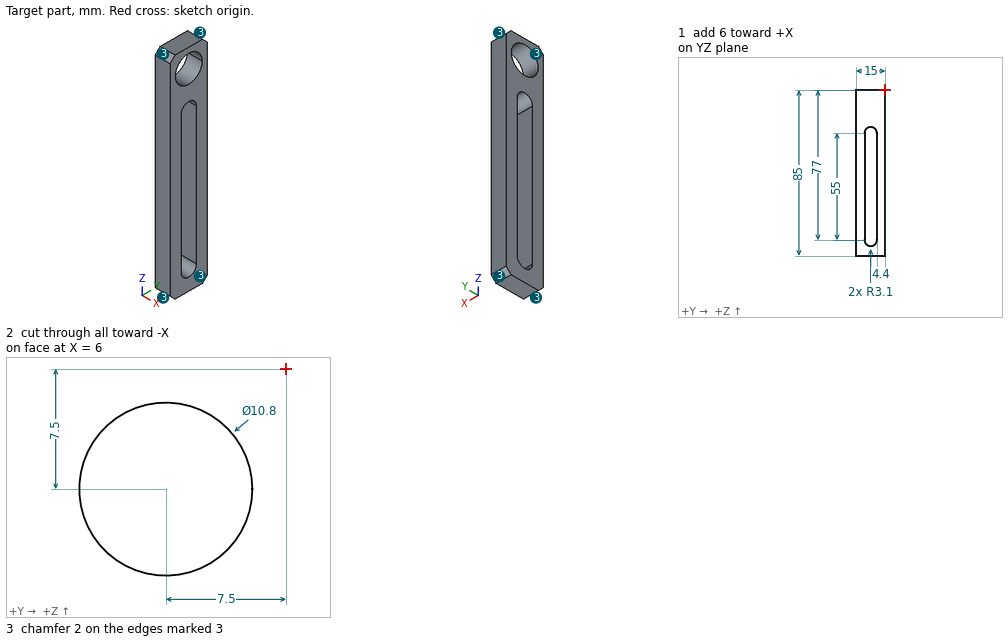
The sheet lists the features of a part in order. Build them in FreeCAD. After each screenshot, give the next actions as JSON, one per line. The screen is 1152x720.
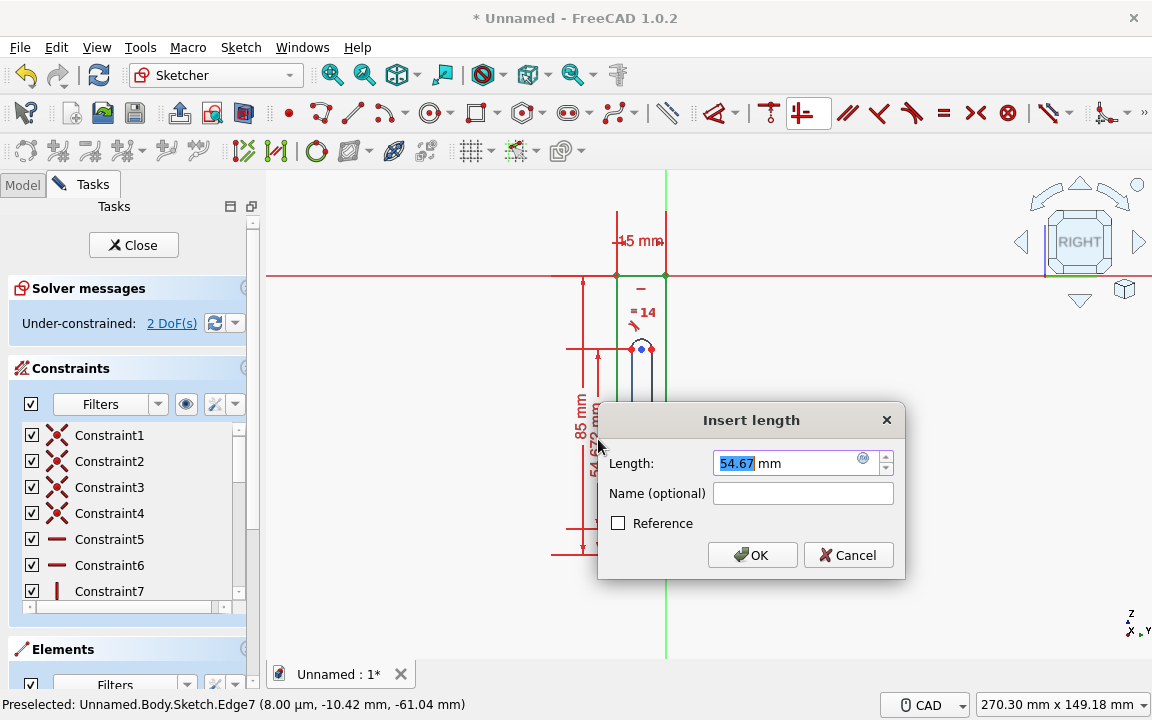
{"action": "type", "text": "55"}
{"action": "key", "text": "Return"}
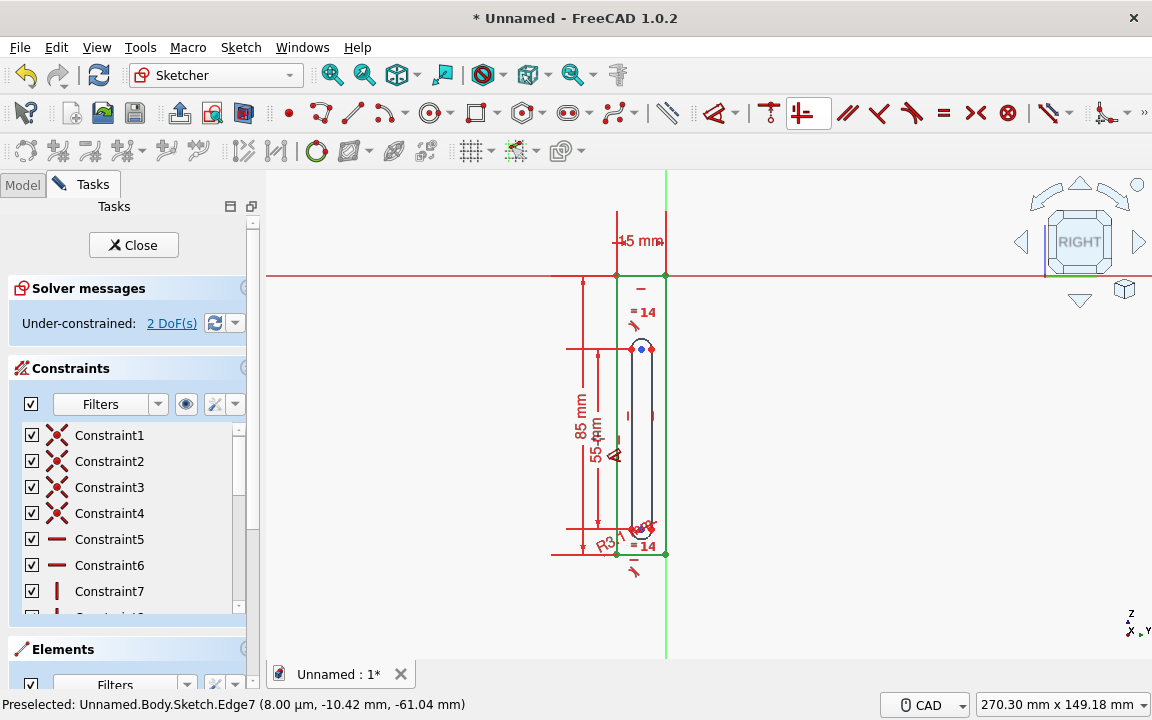
{"action": "left_click", "coordinate": [632, 529]}
{"action": "left_click", "coordinate": [700, 403]}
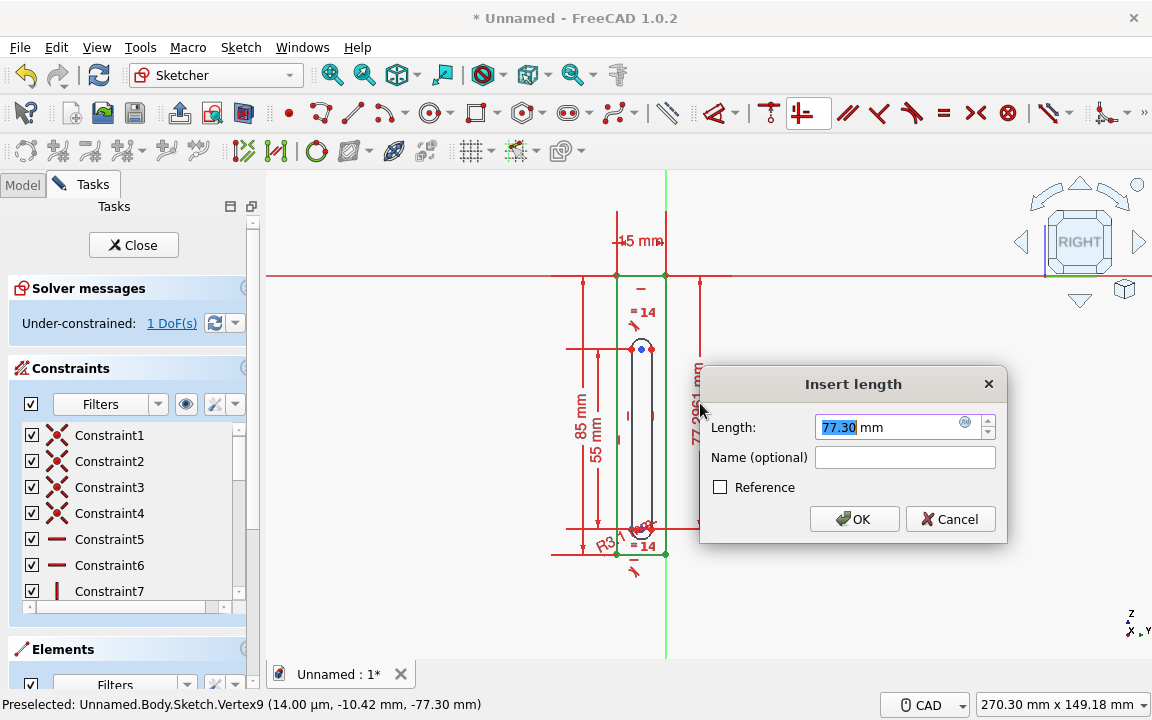
{"action": "type", "text": "77"}
{"action": "key", "text": "Return"}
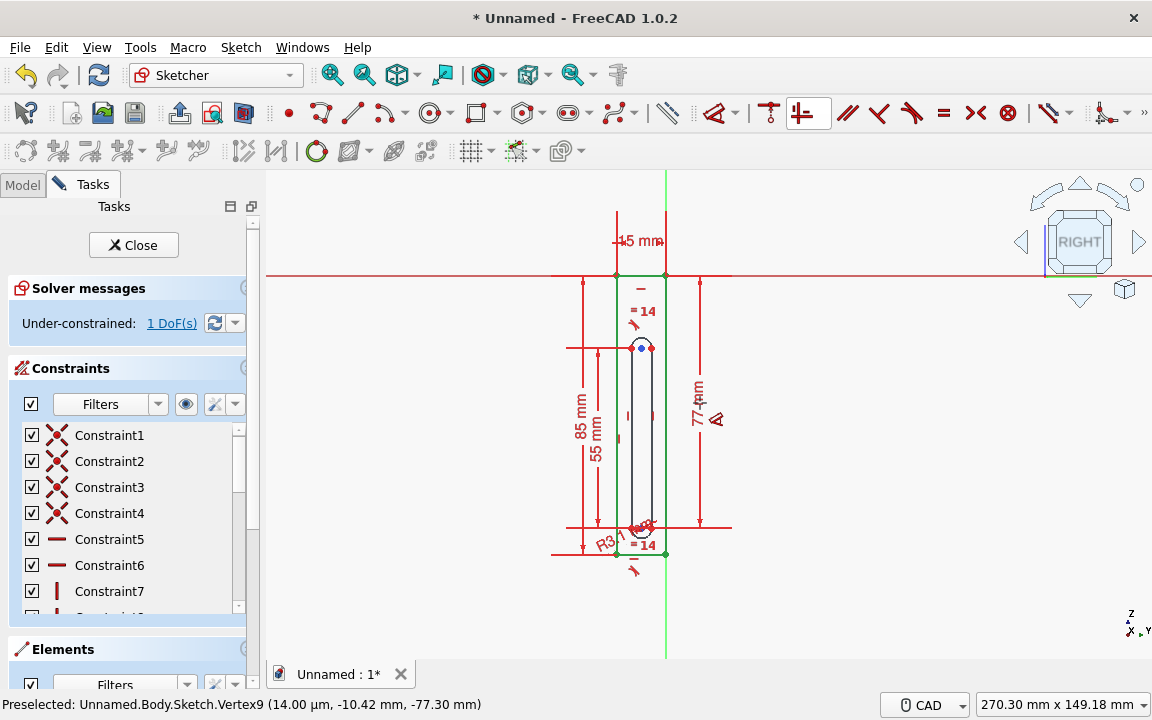
{"action": "scroll", "coordinate": [652, 528], "scroll_direction": "up", "scroll_amount": 6}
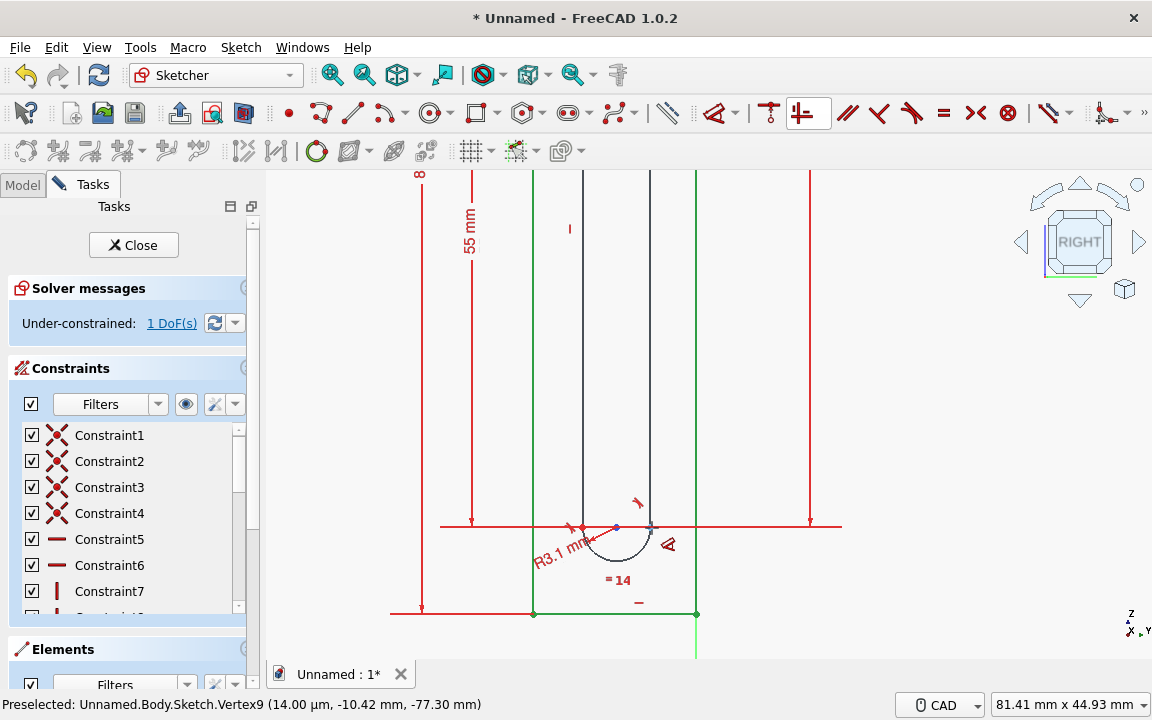
{"action": "left_click", "coordinate": [650, 527]}
{"action": "left_click", "coordinate": [673, 561]}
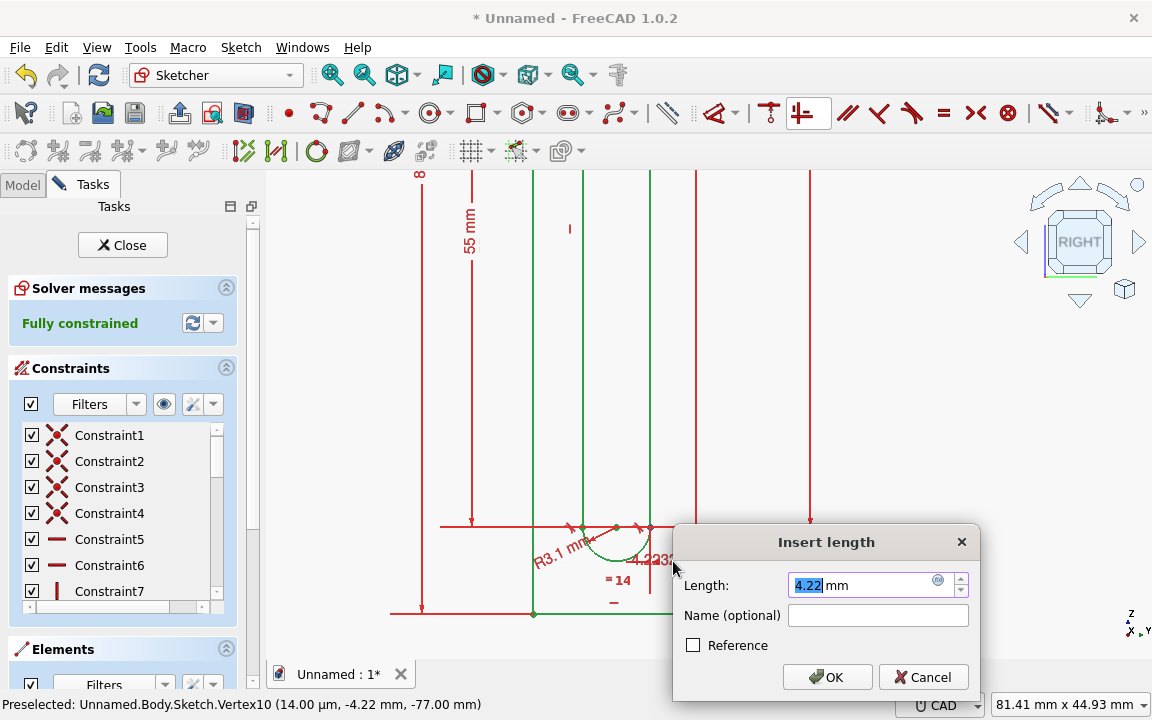
{"action": "type", "text": "4.4"}
{"action": "key", "text": "Return"}
{"action": "key", "text": "Escape"}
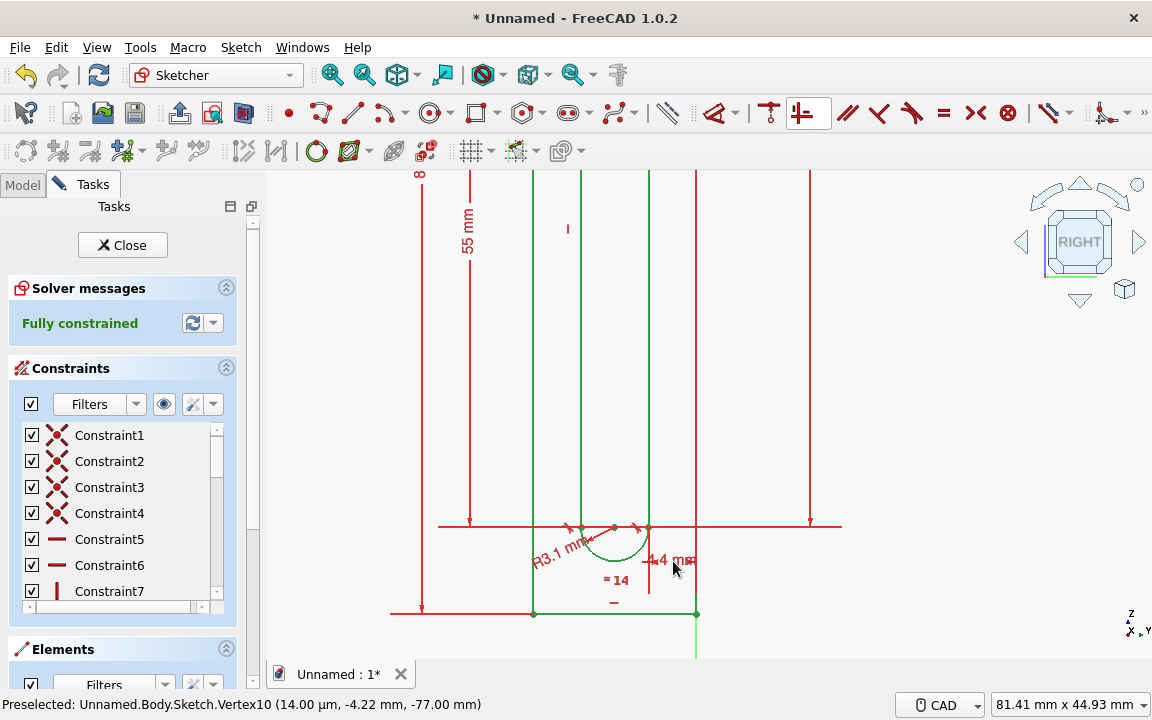
{"action": "left_click", "coordinate": [123, 245]}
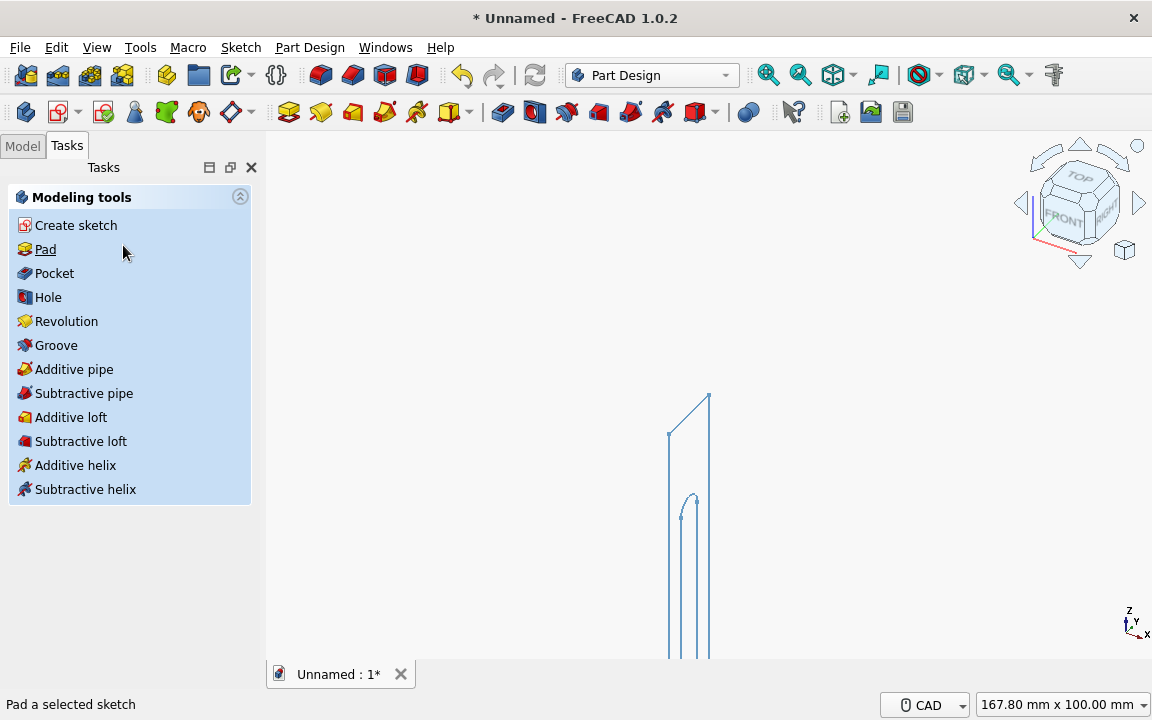
{"action": "left_click", "coordinate": [290, 112]}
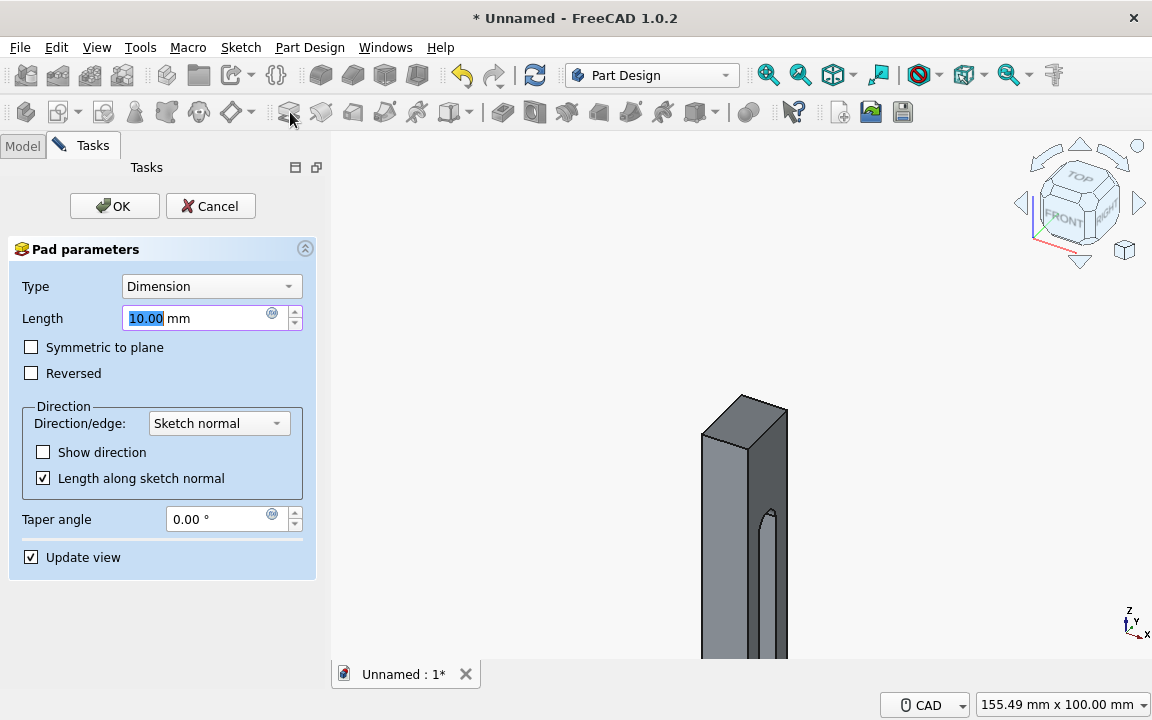
{"action": "type", "text": "6"}
{"action": "key", "text": "Tab"}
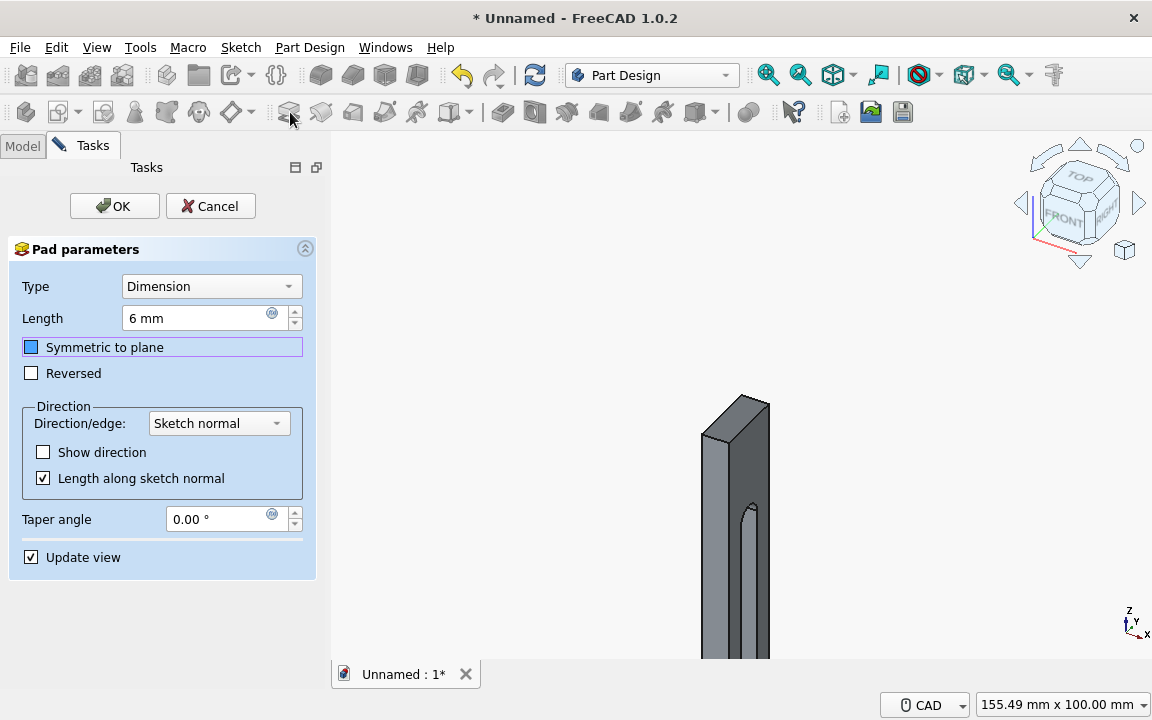
{"action": "left_click", "coordinate": [115, 206]}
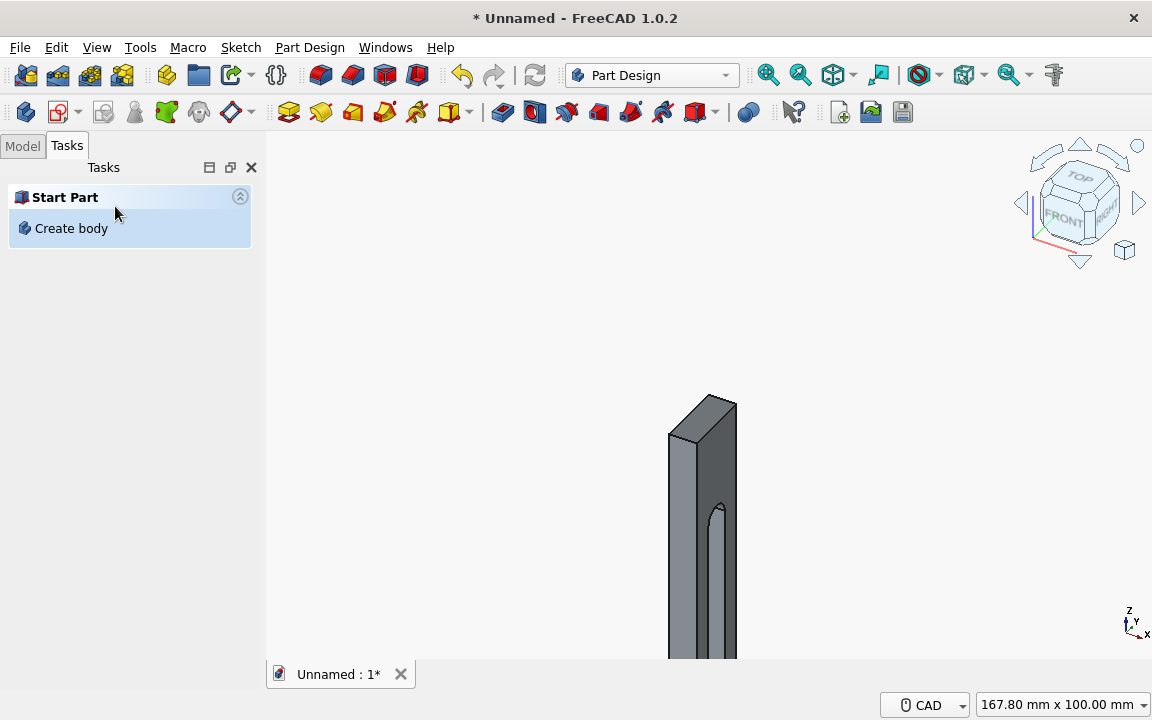
{"action": "left_click", "coordinate": [770, 76]}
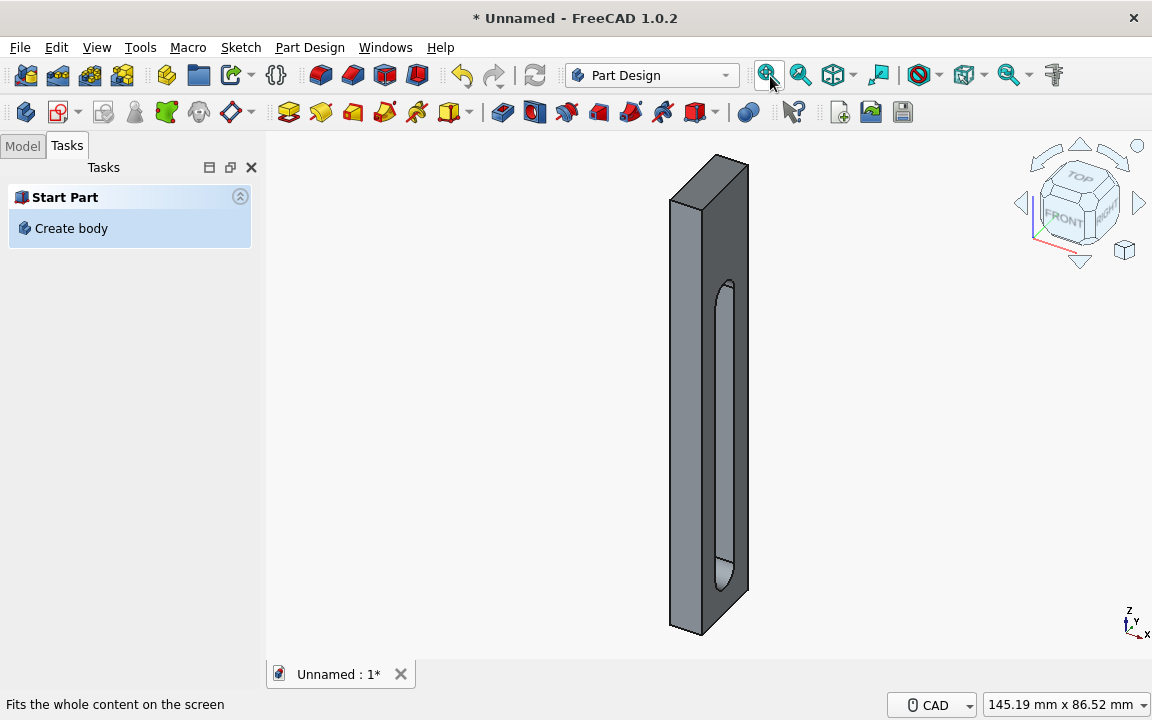
{"action": "left_click", "coordinate": [725, 217]}